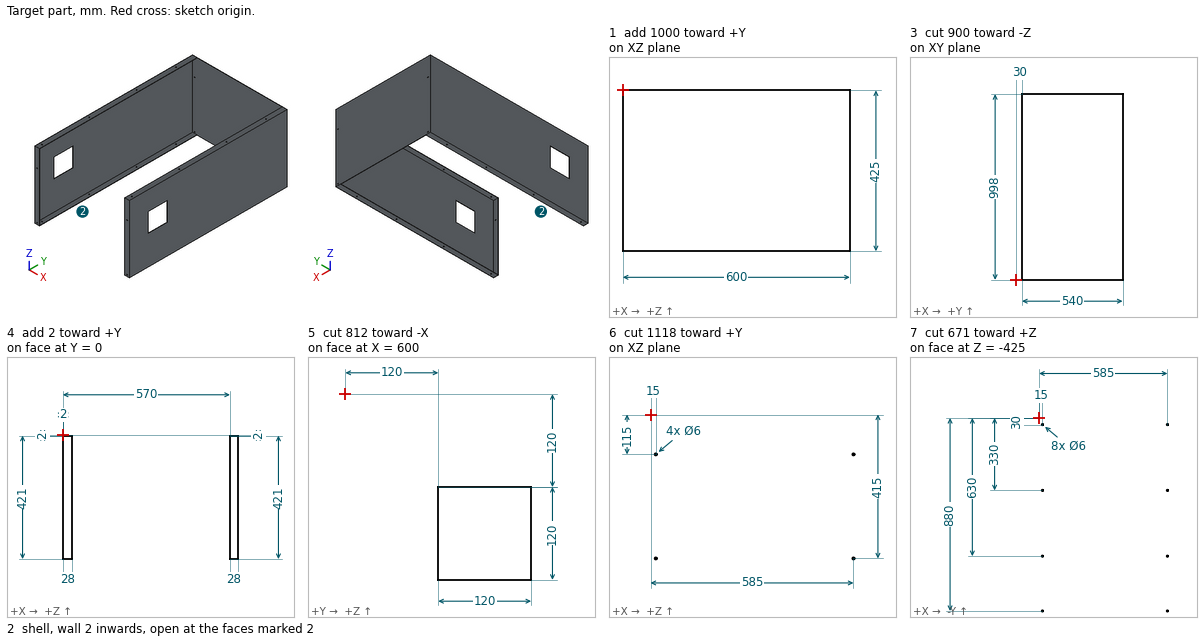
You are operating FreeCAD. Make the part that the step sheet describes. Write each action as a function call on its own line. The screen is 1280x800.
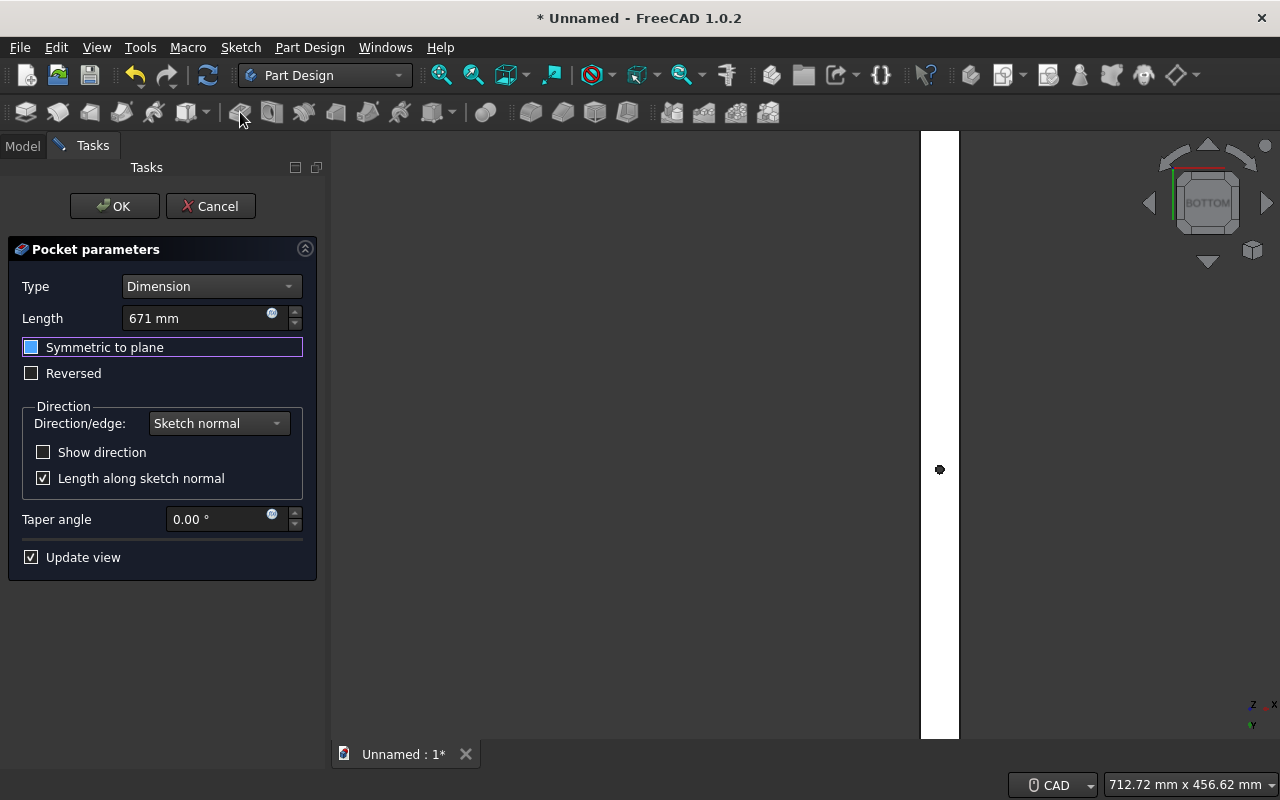
click(115, 206)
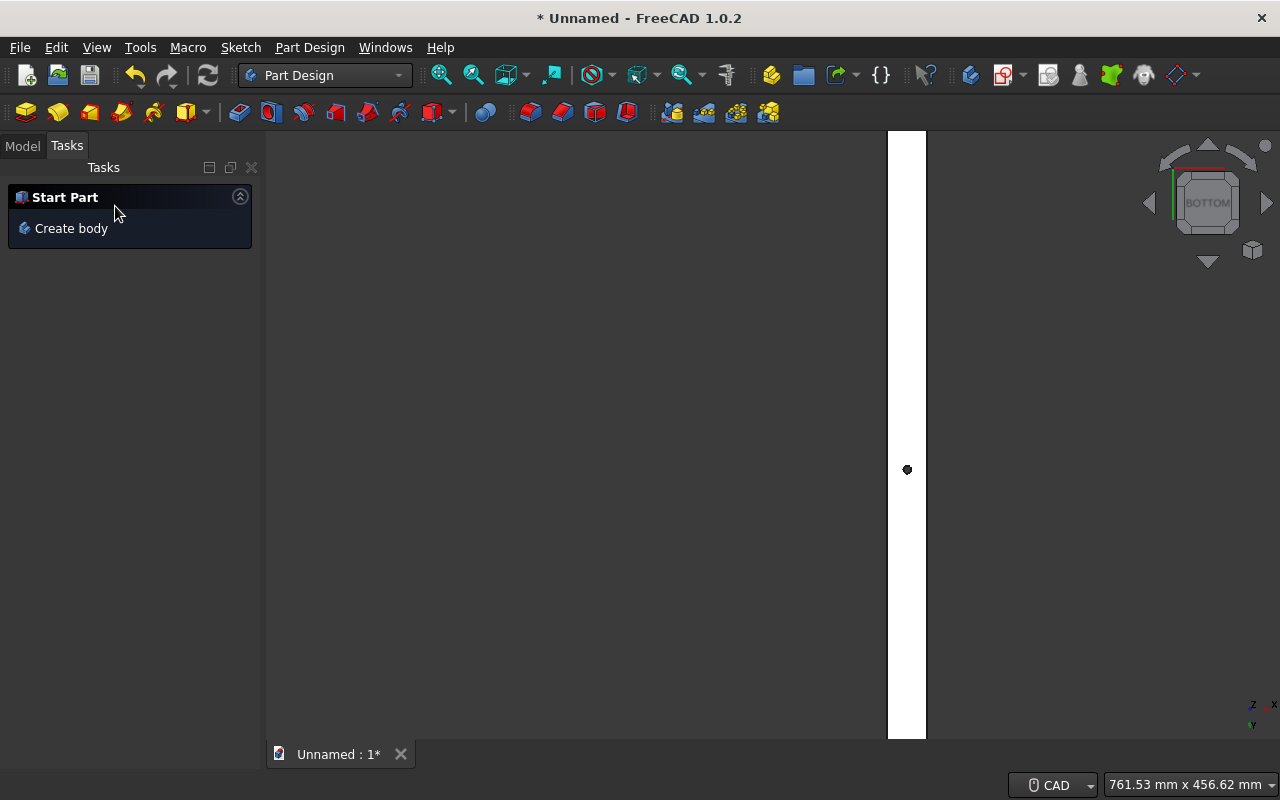
key(0)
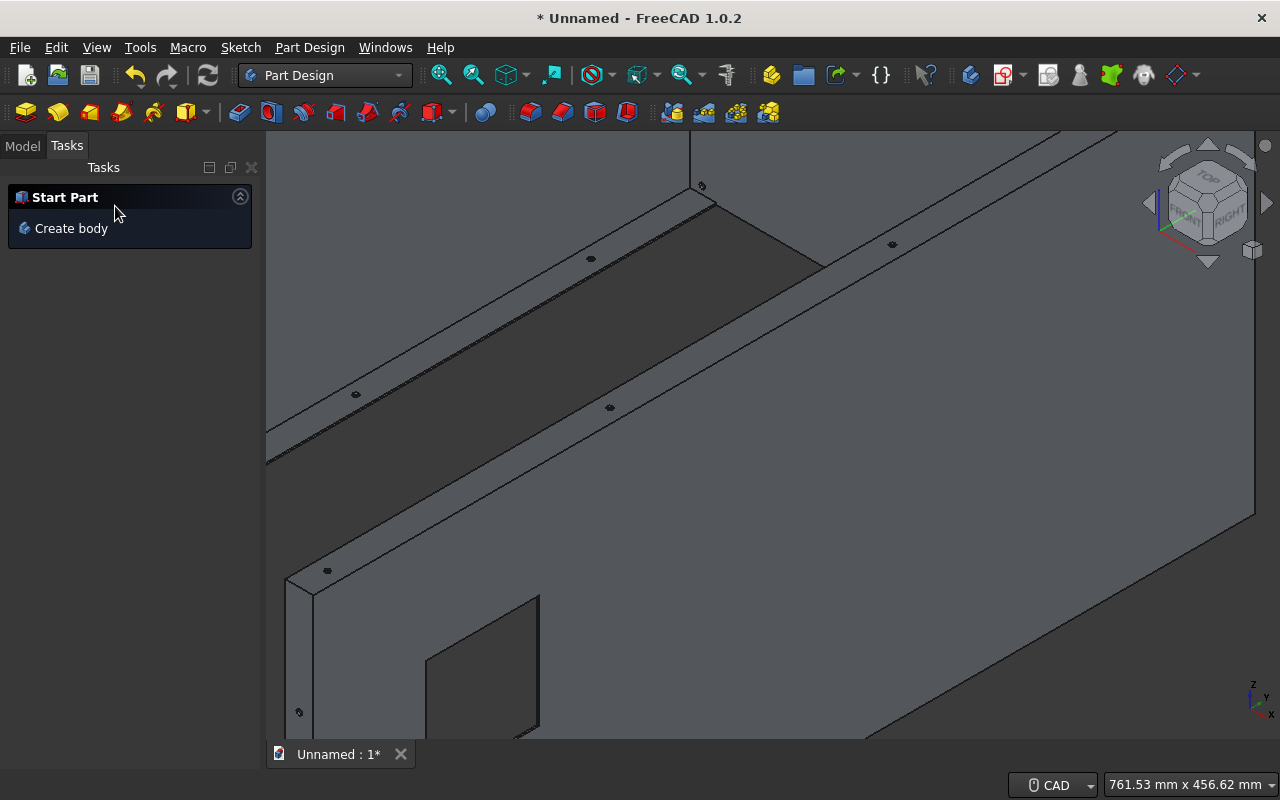
click(442, 76)